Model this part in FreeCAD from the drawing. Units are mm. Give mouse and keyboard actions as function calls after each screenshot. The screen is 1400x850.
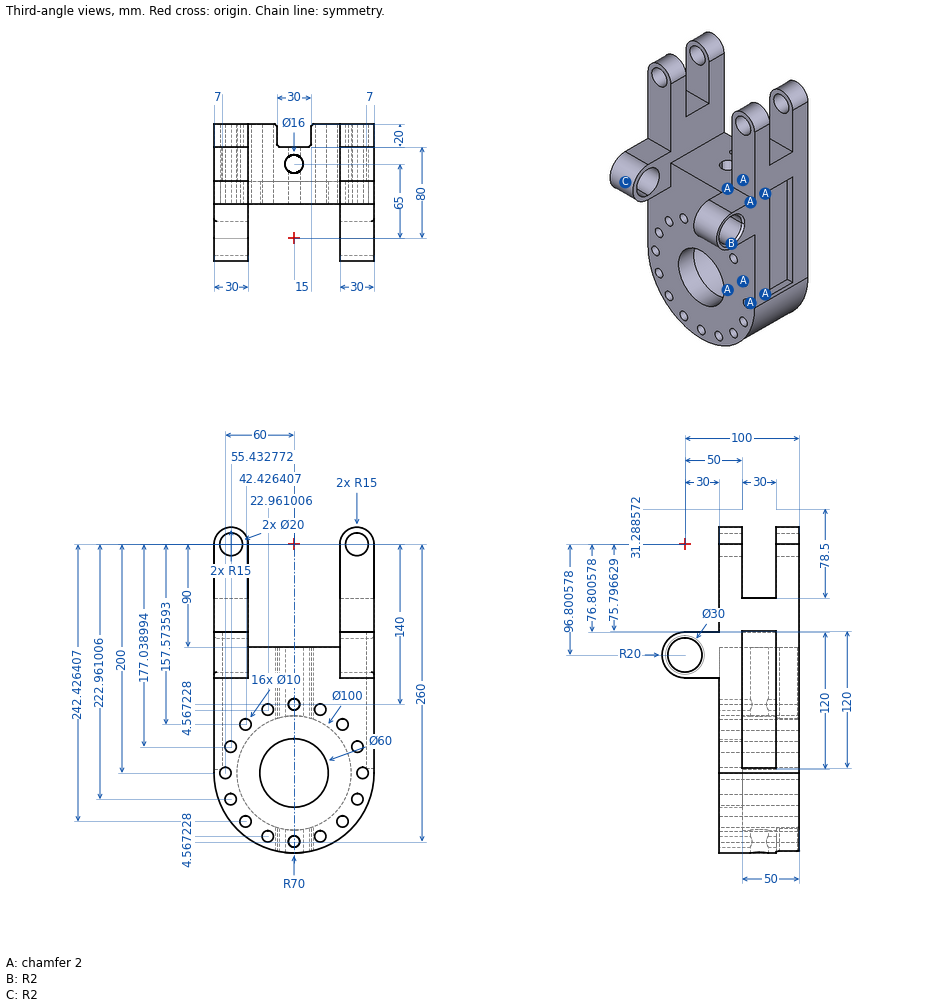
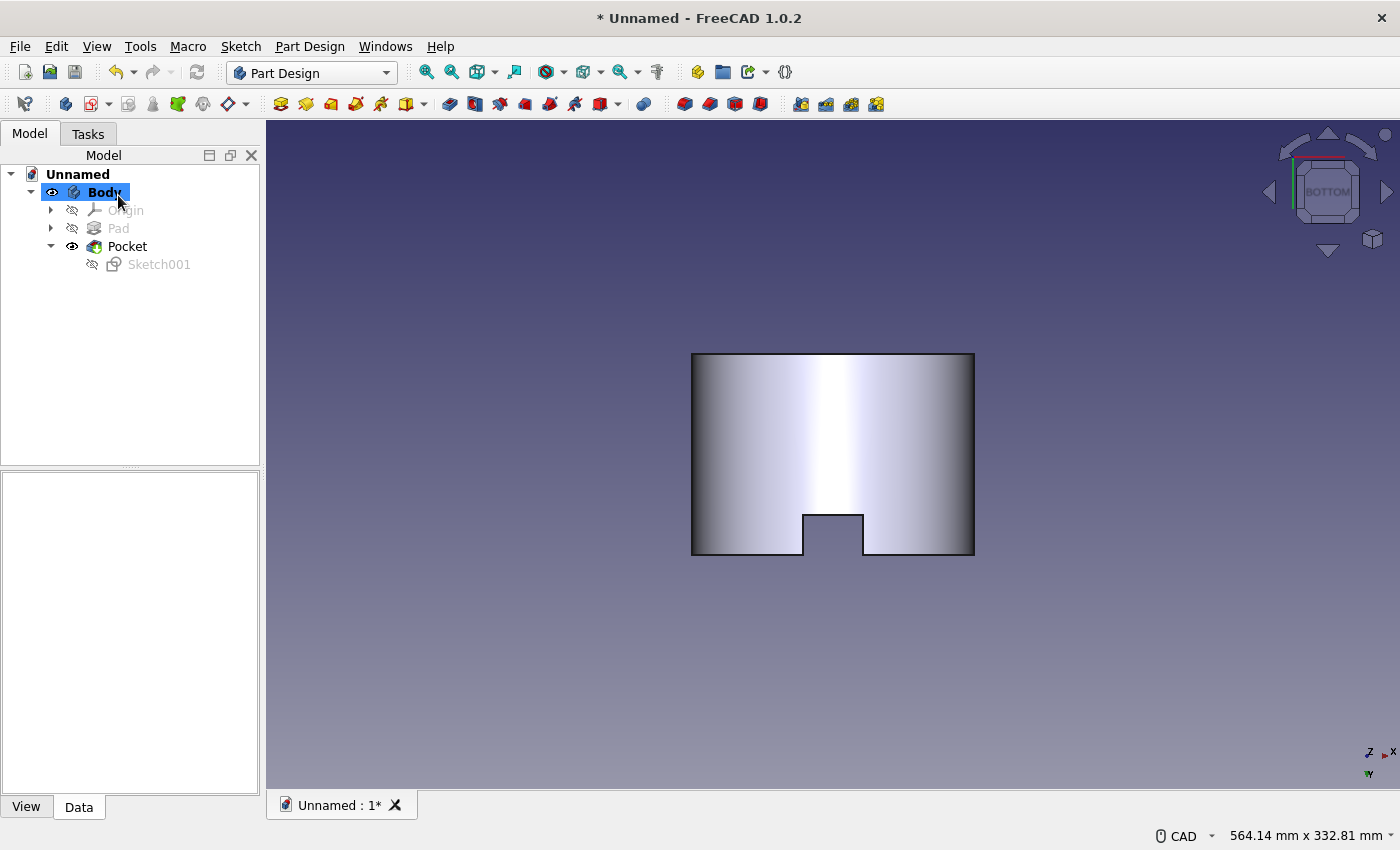
key(v)
key(f)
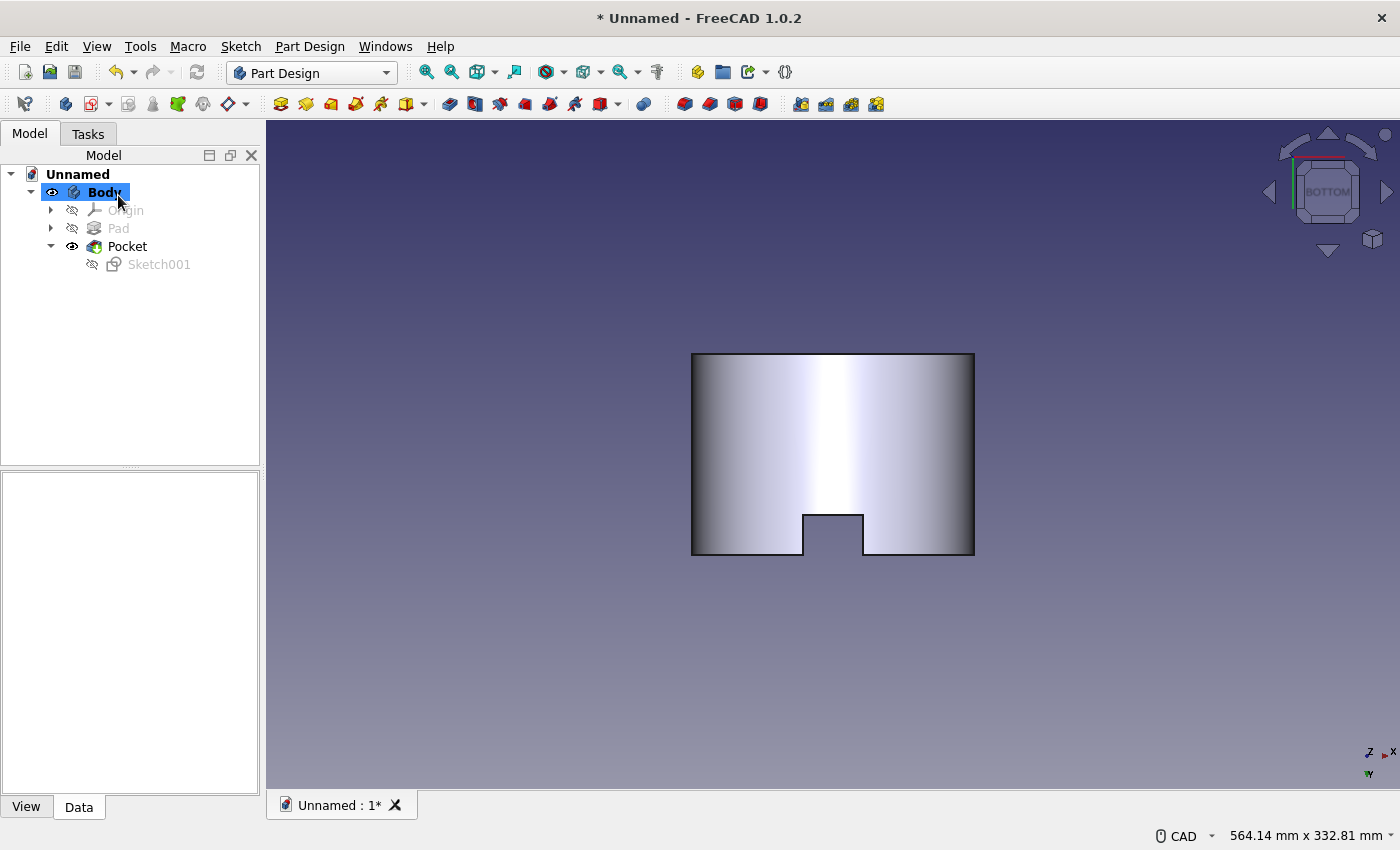
key(4)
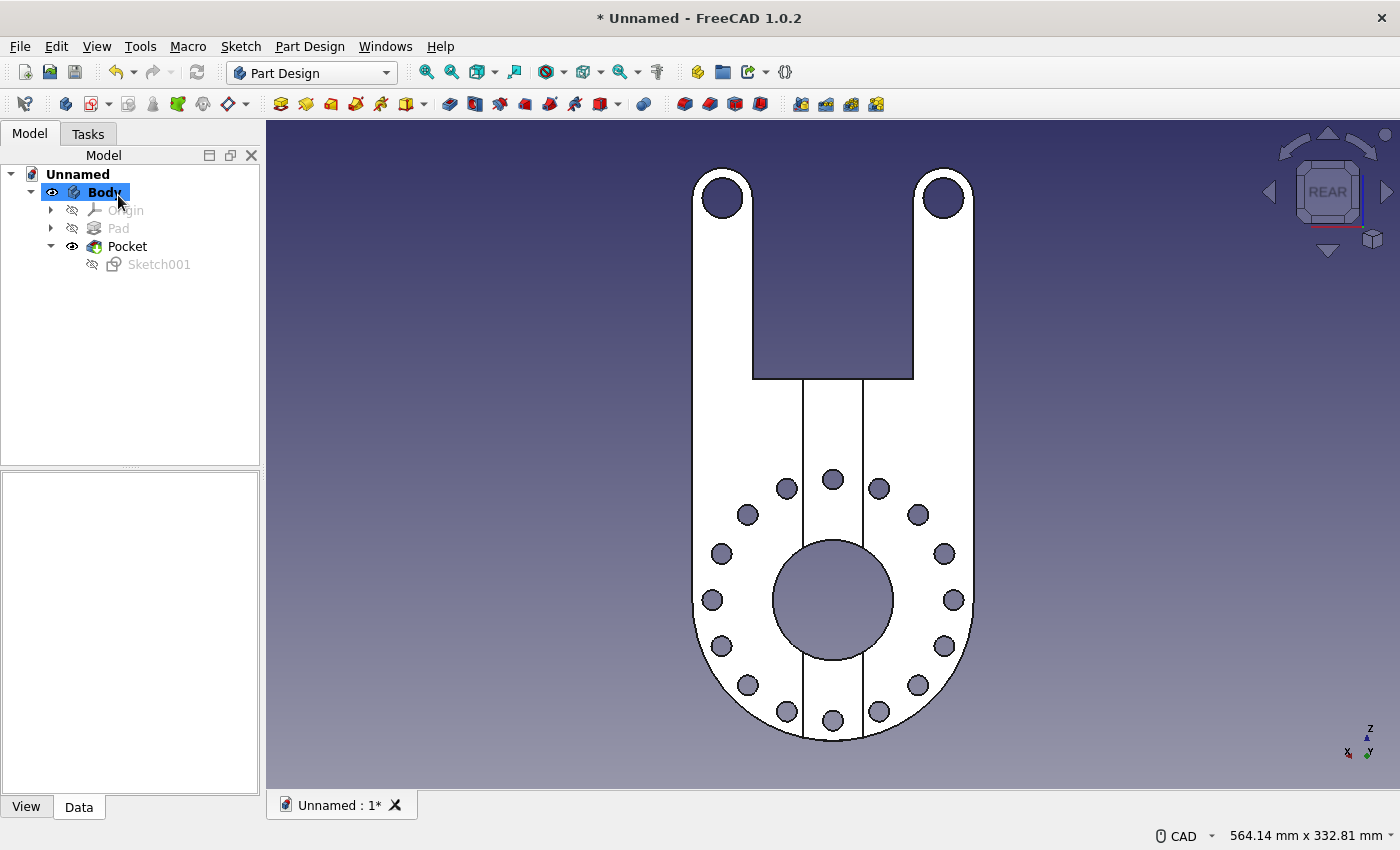
click(803, 694)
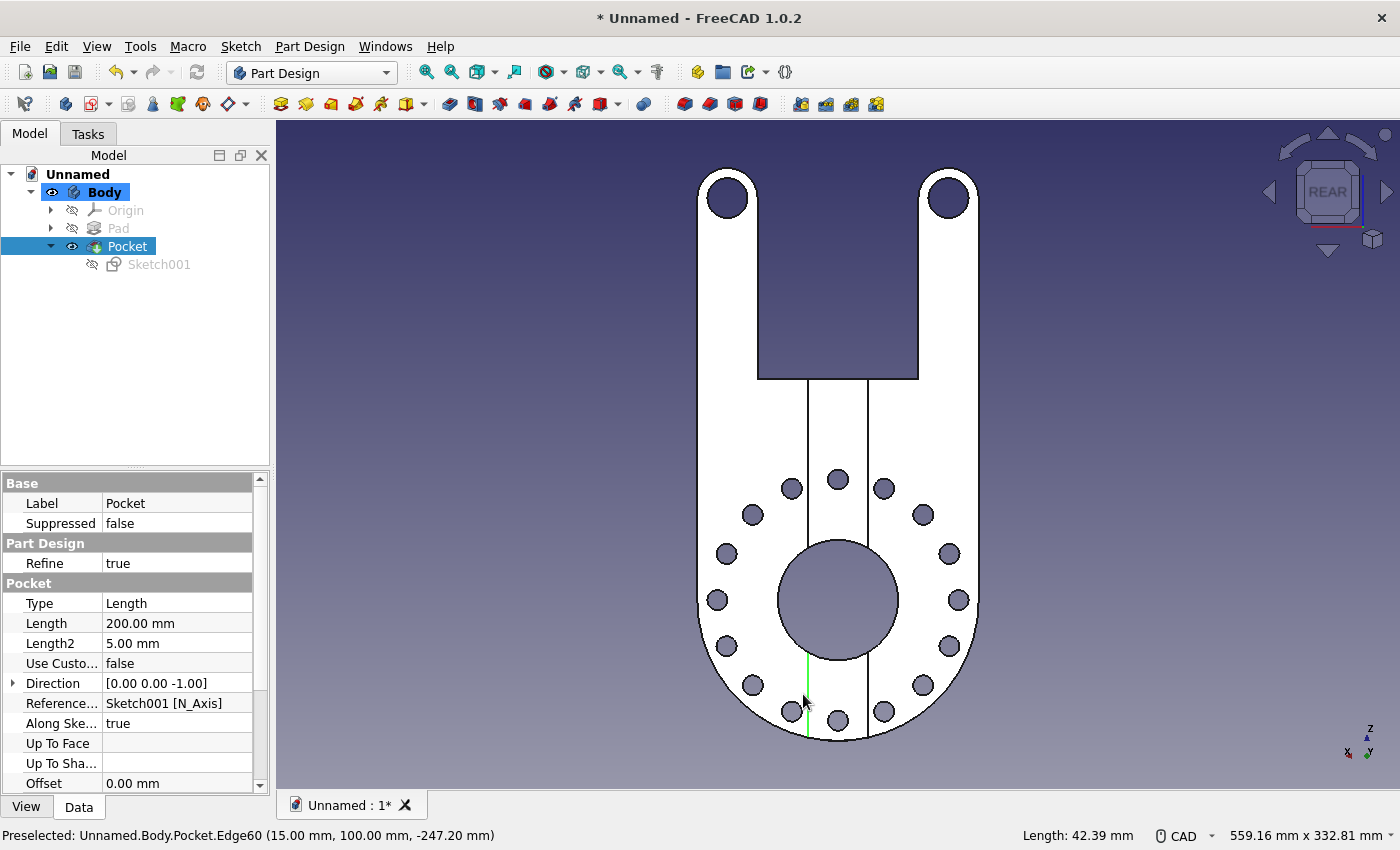
click(868, 694, ctrl)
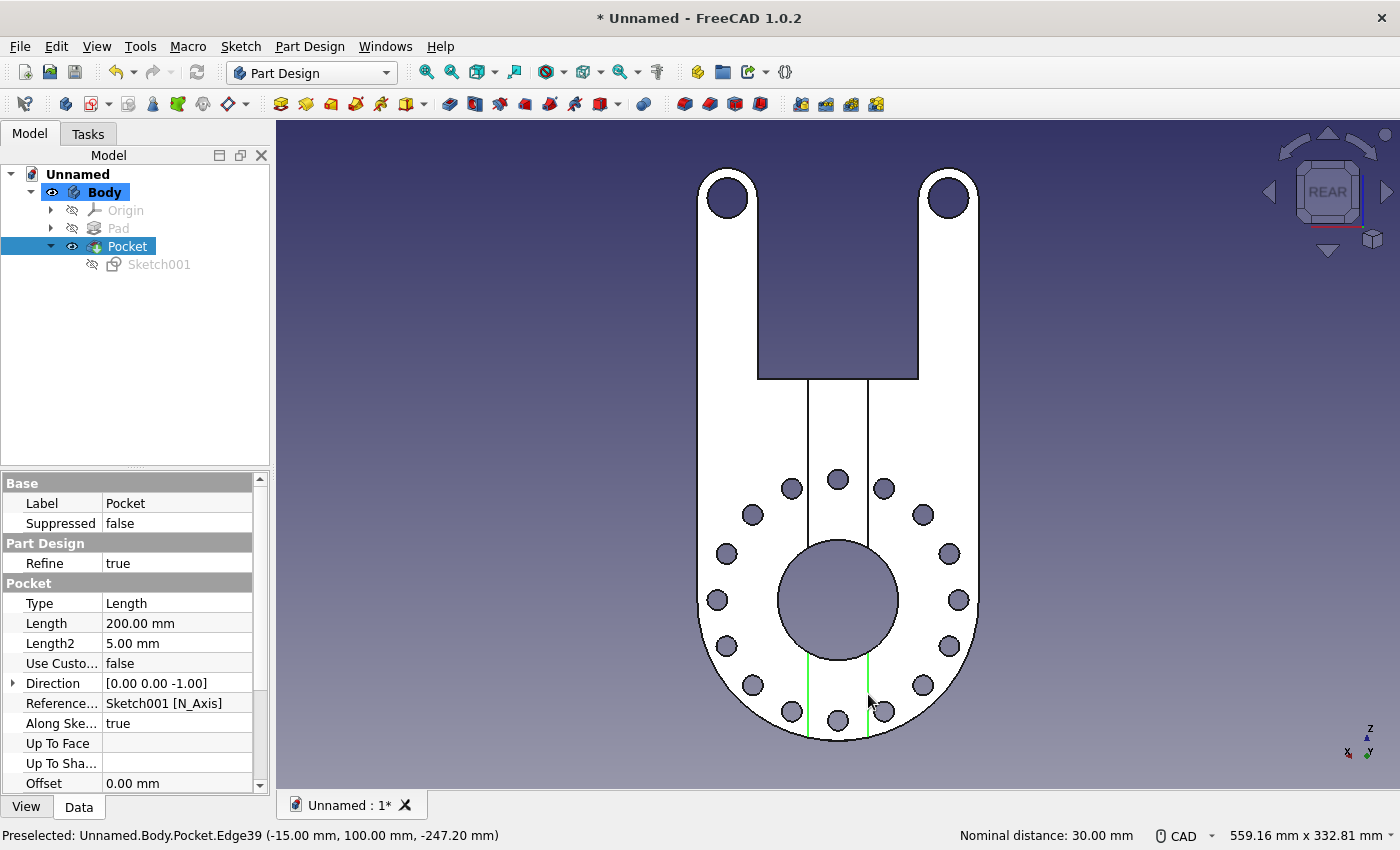
click(808, 462, ctrl)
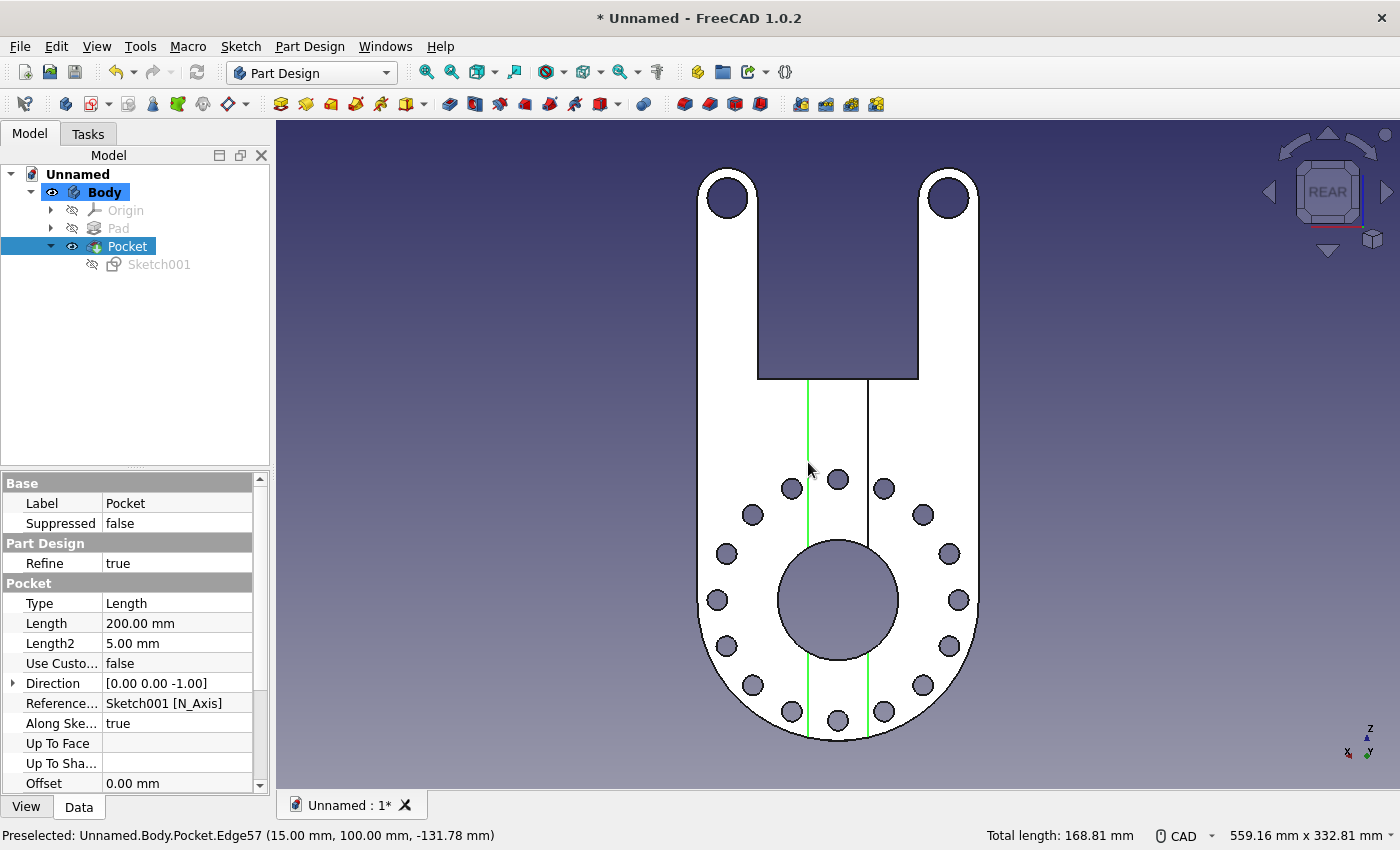
click(868, 462, ctrl)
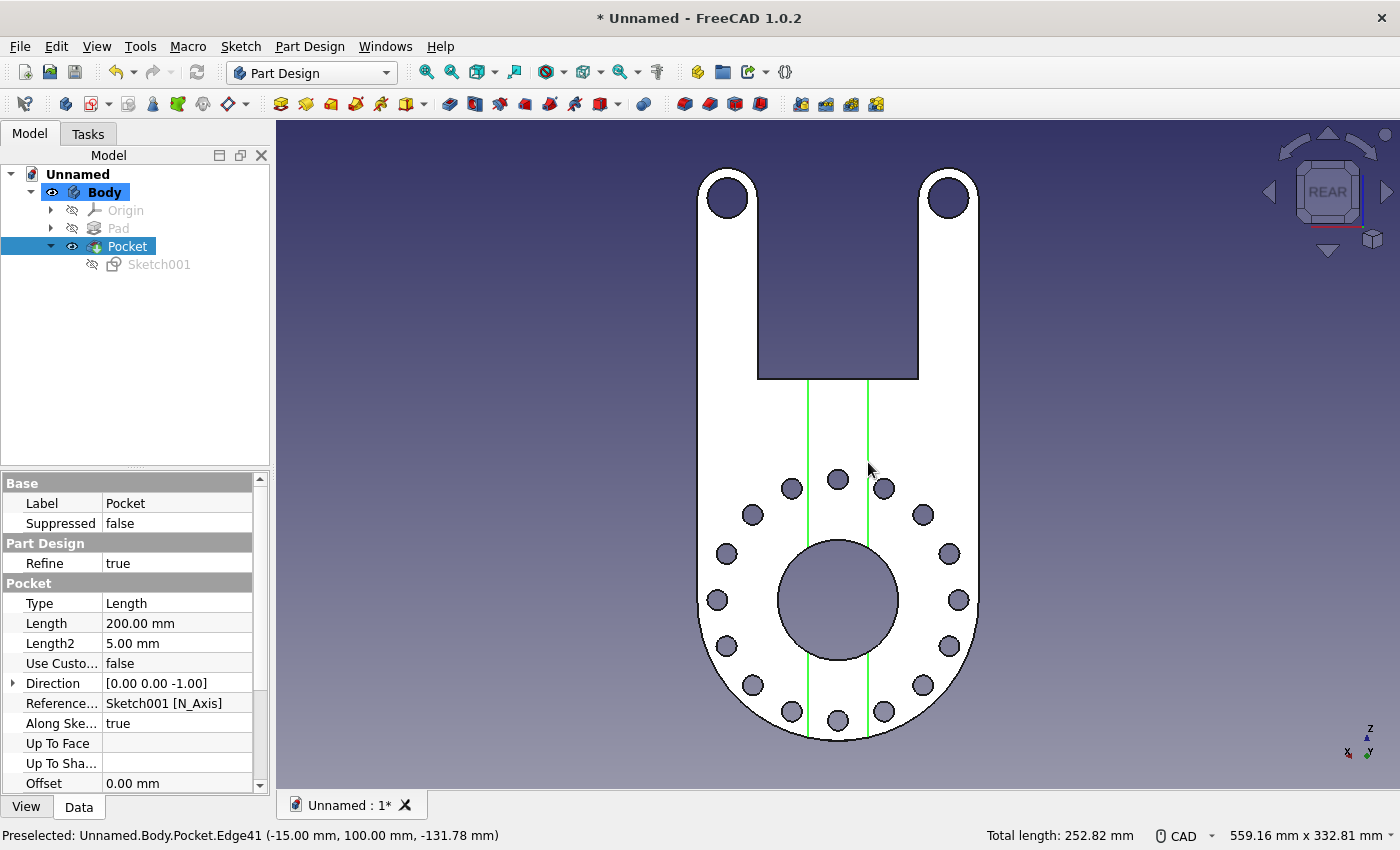
key(6)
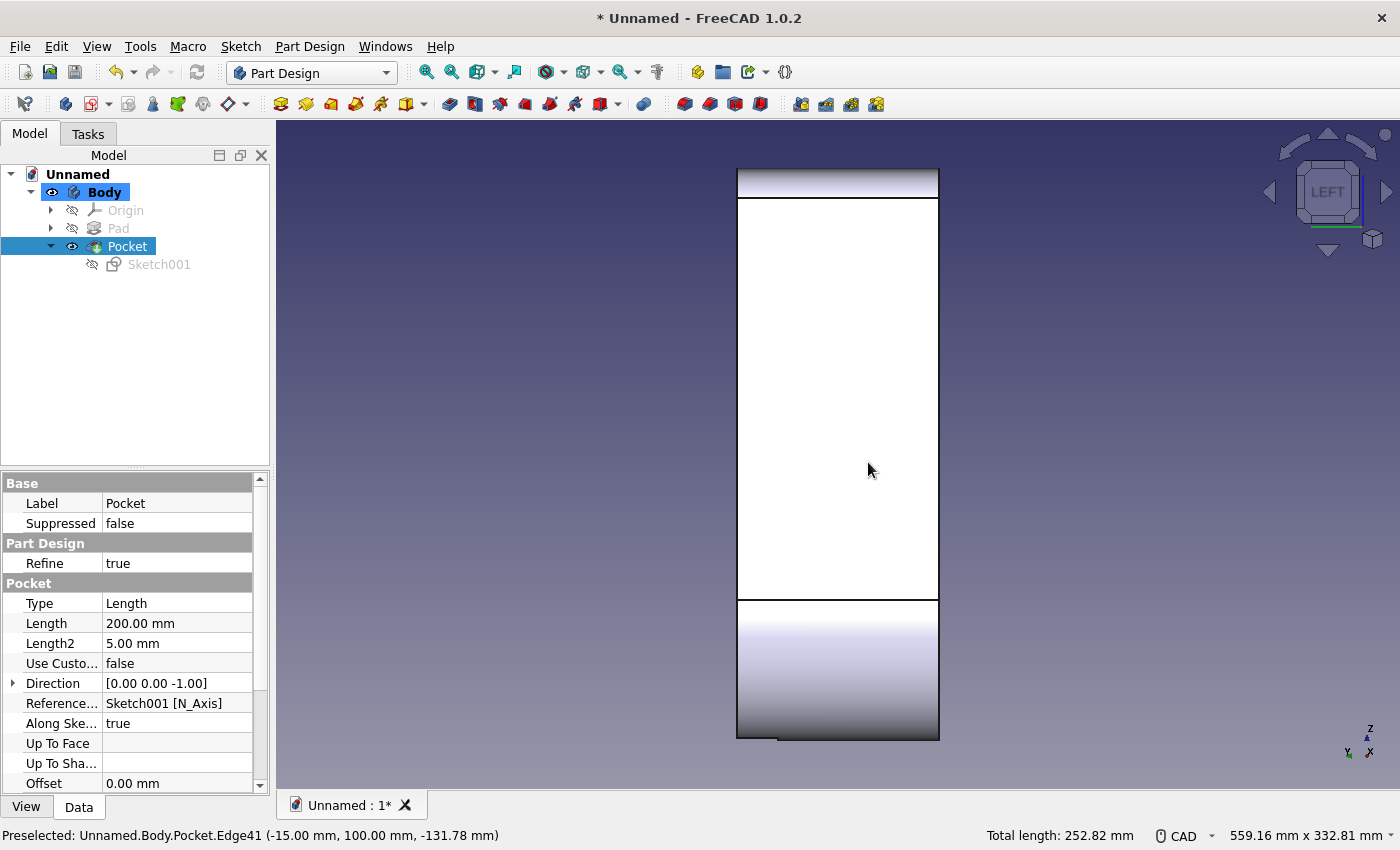
key(v)
key(3)